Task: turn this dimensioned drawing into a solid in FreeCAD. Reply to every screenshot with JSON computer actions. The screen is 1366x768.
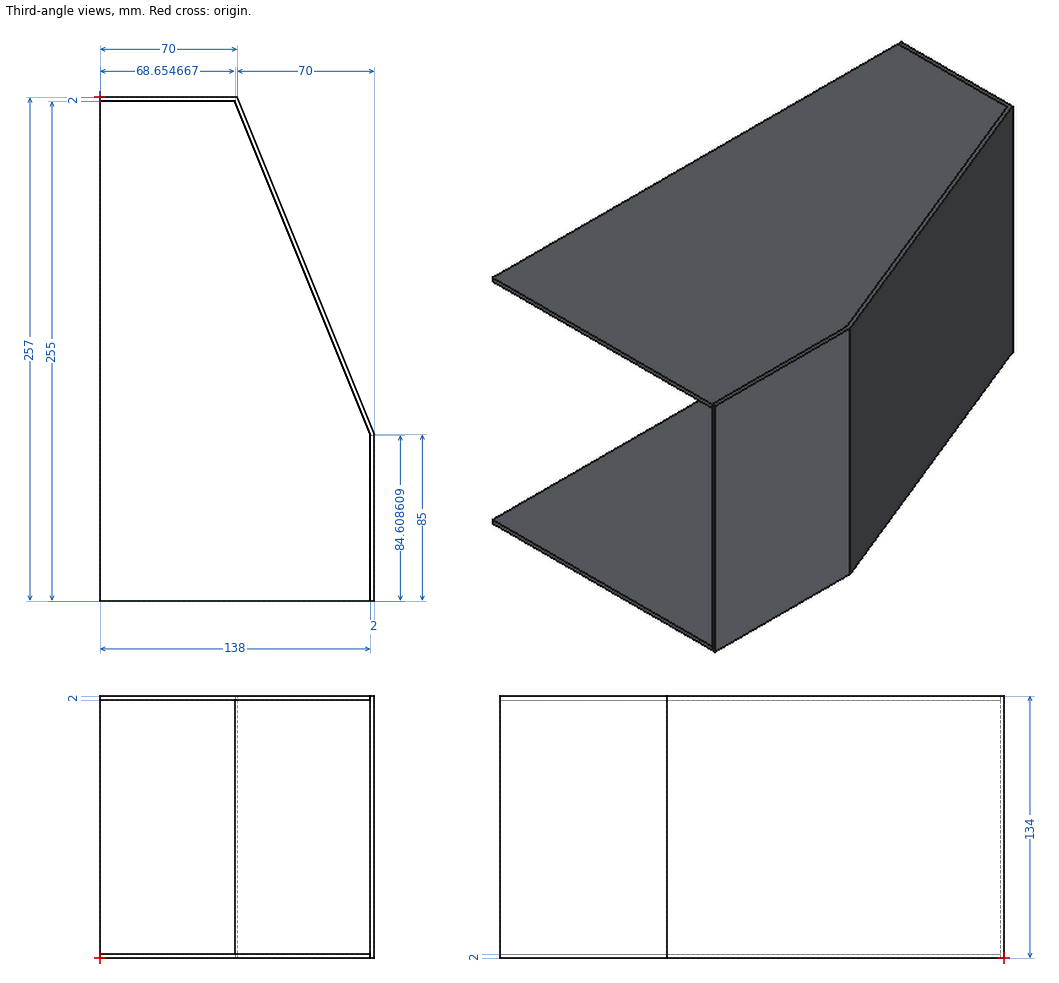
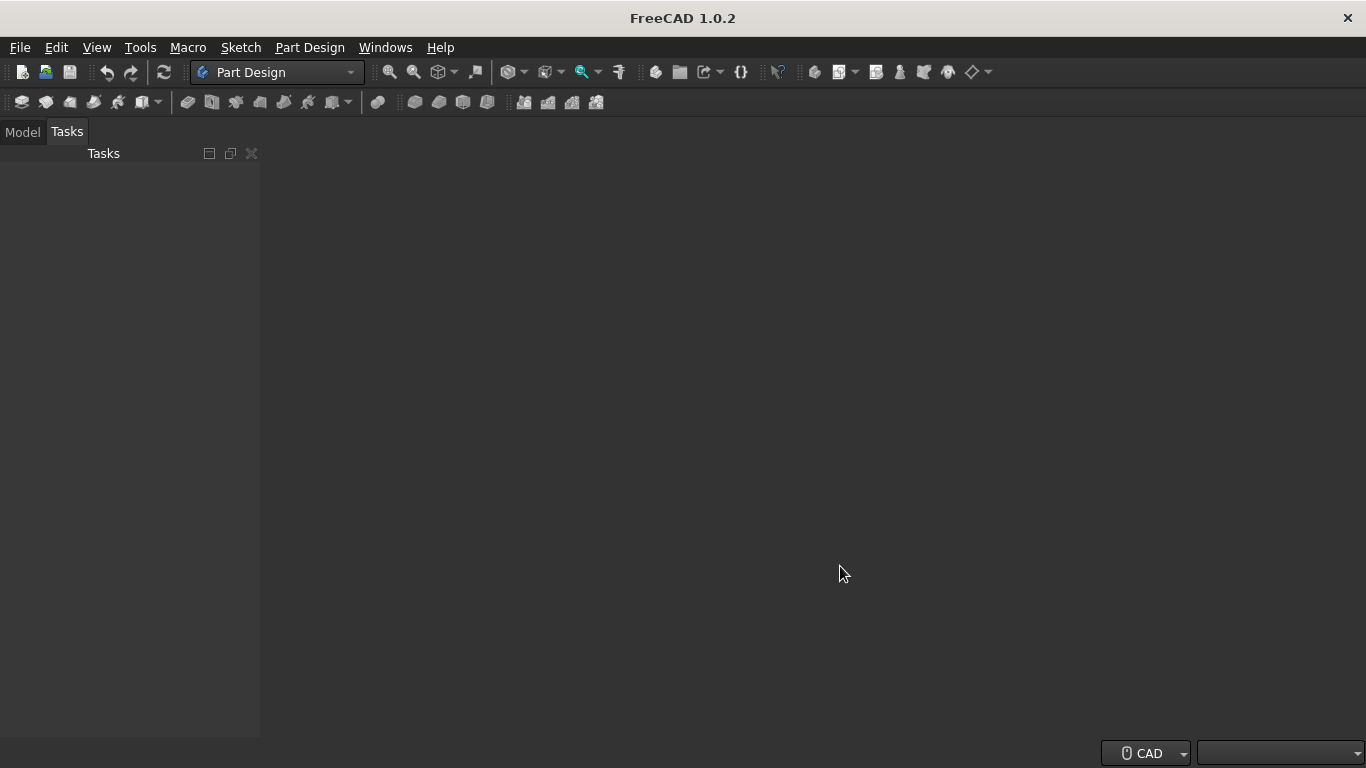
{"action": "left_click", "coordinate": [22, 72]}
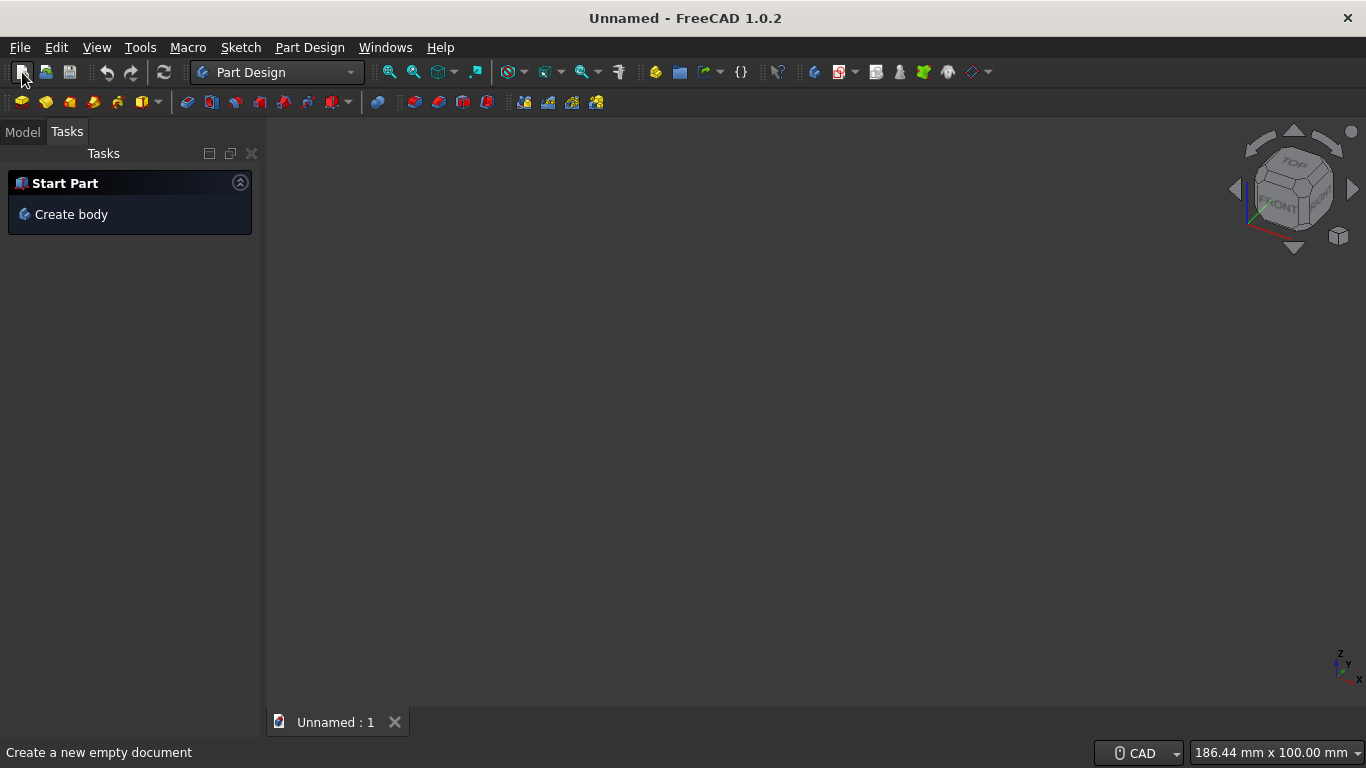
{"action": "left_click", "coordinate": [840, 72]}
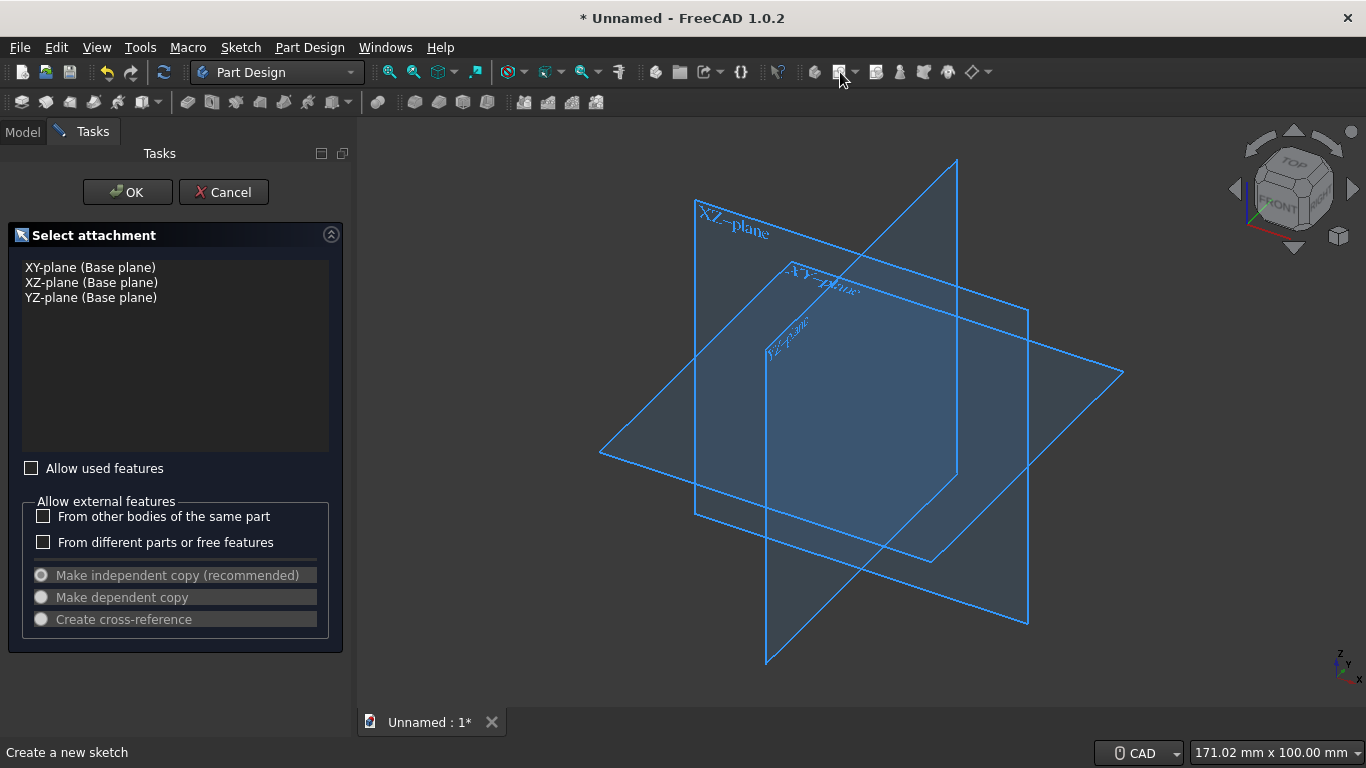
{"action": "left_click", "coordinate": [82, 268]}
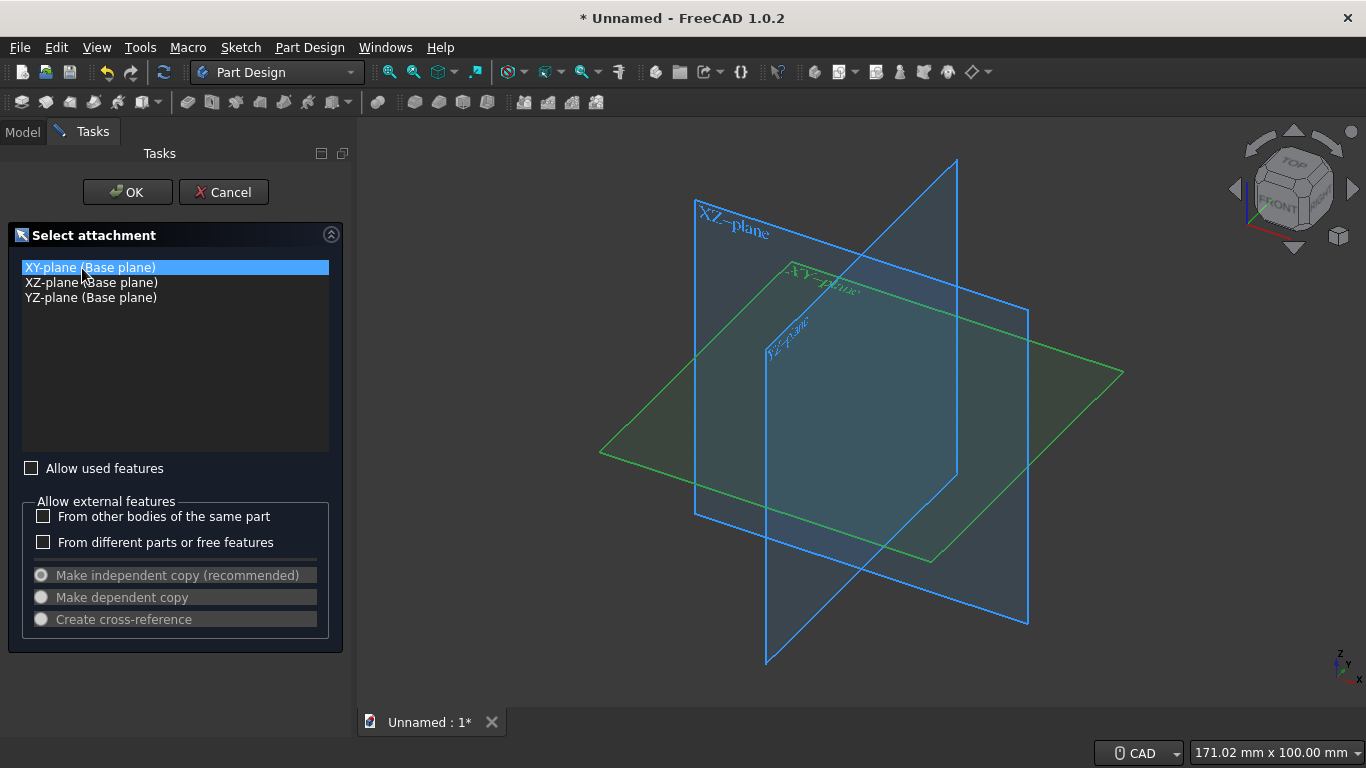
{"action": "left_click", "coordinate": [128, 192]}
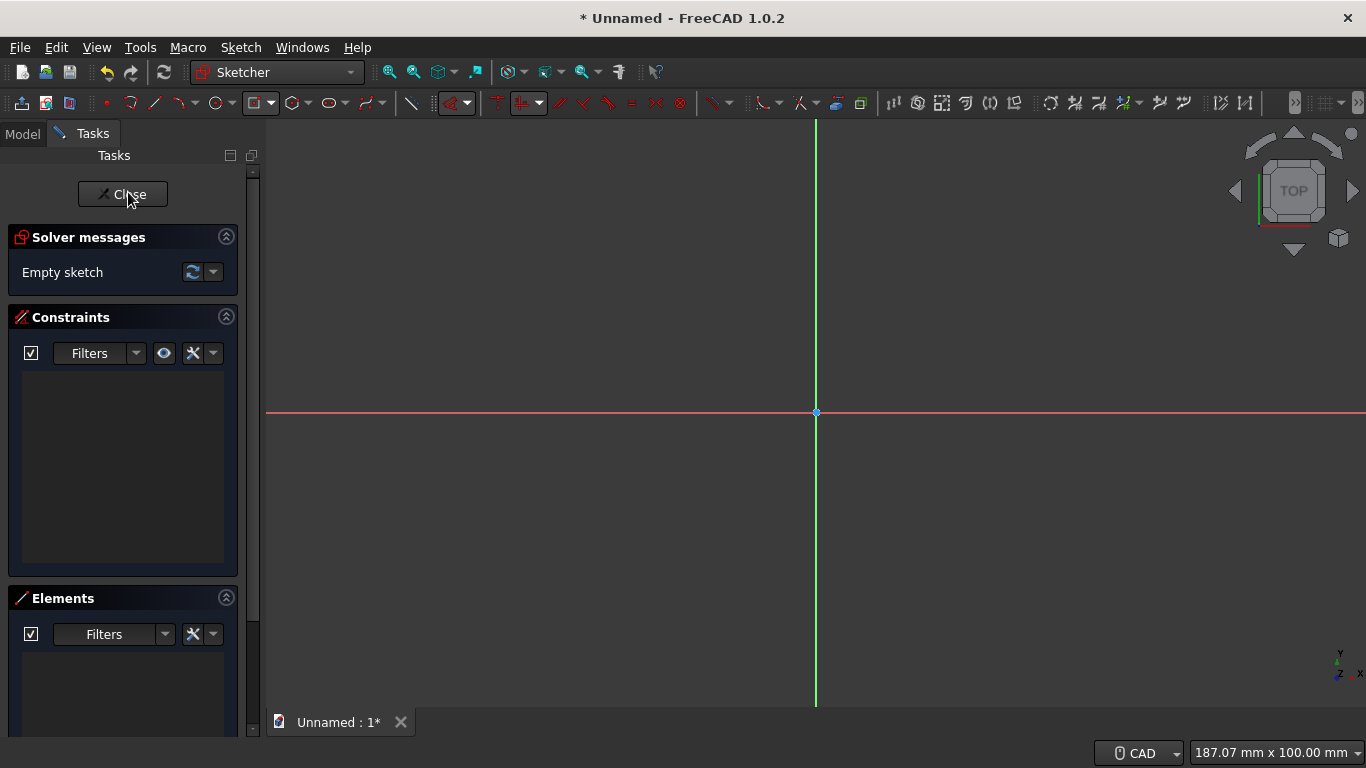
{"action": "scroll", "coordinate": [590, 166], "scroll_direction": "down", "scroll_amount": 7}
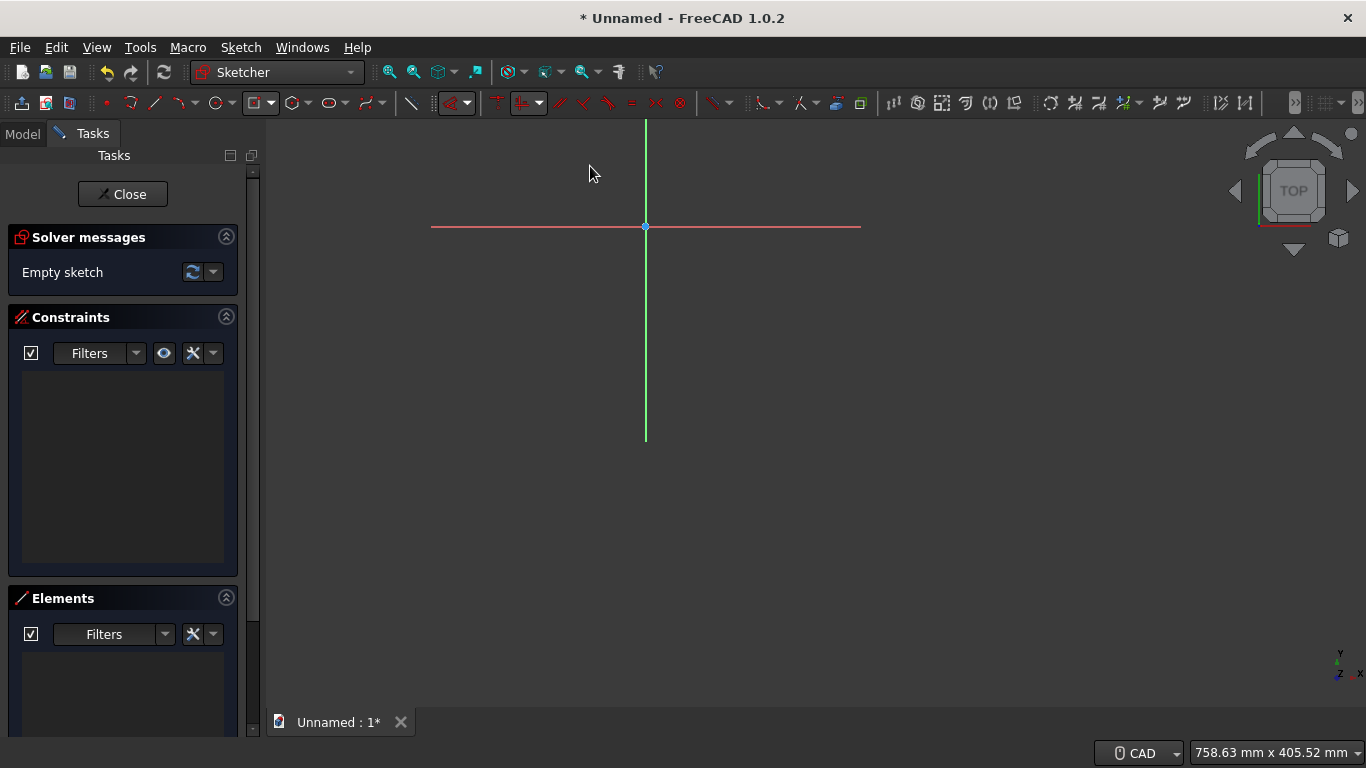
{"action": "key", "text": "g m"}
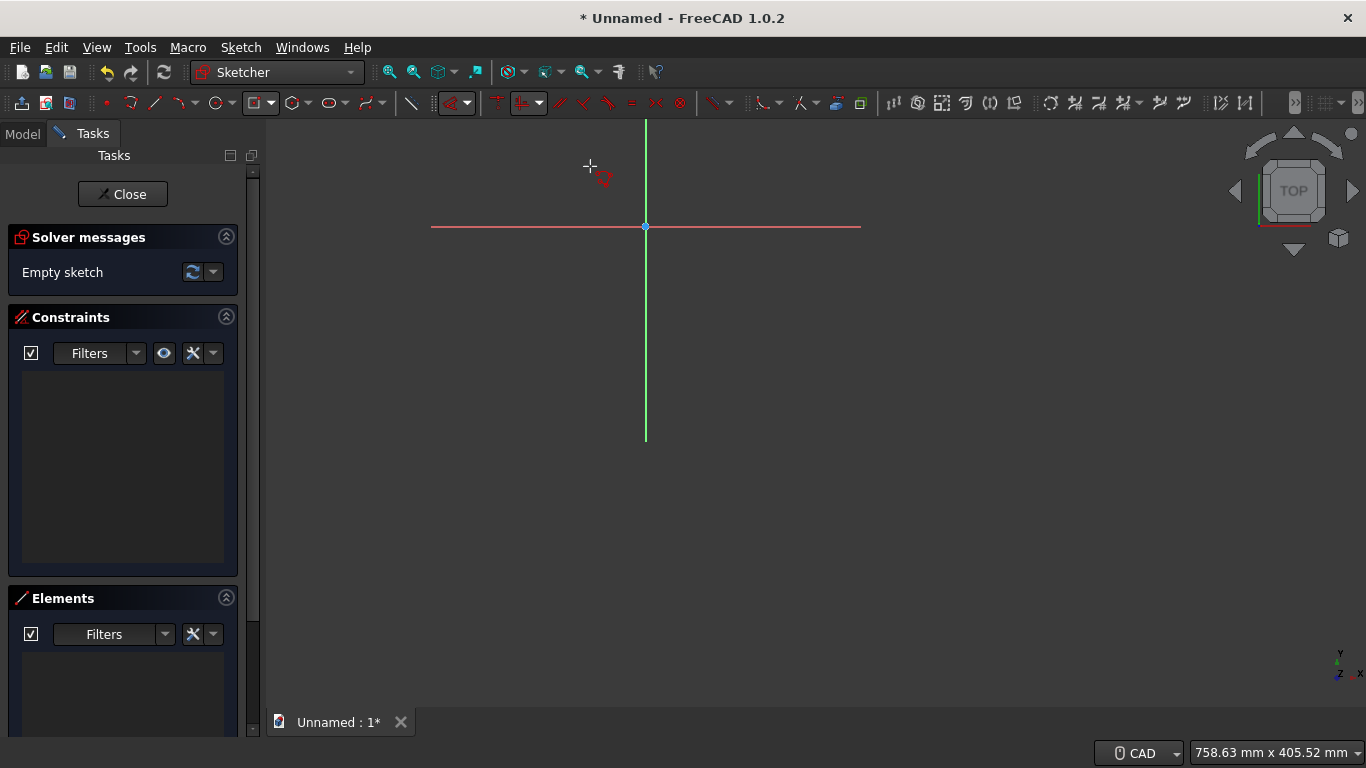
{"action": "left_click", "coordinate": [646, 227]}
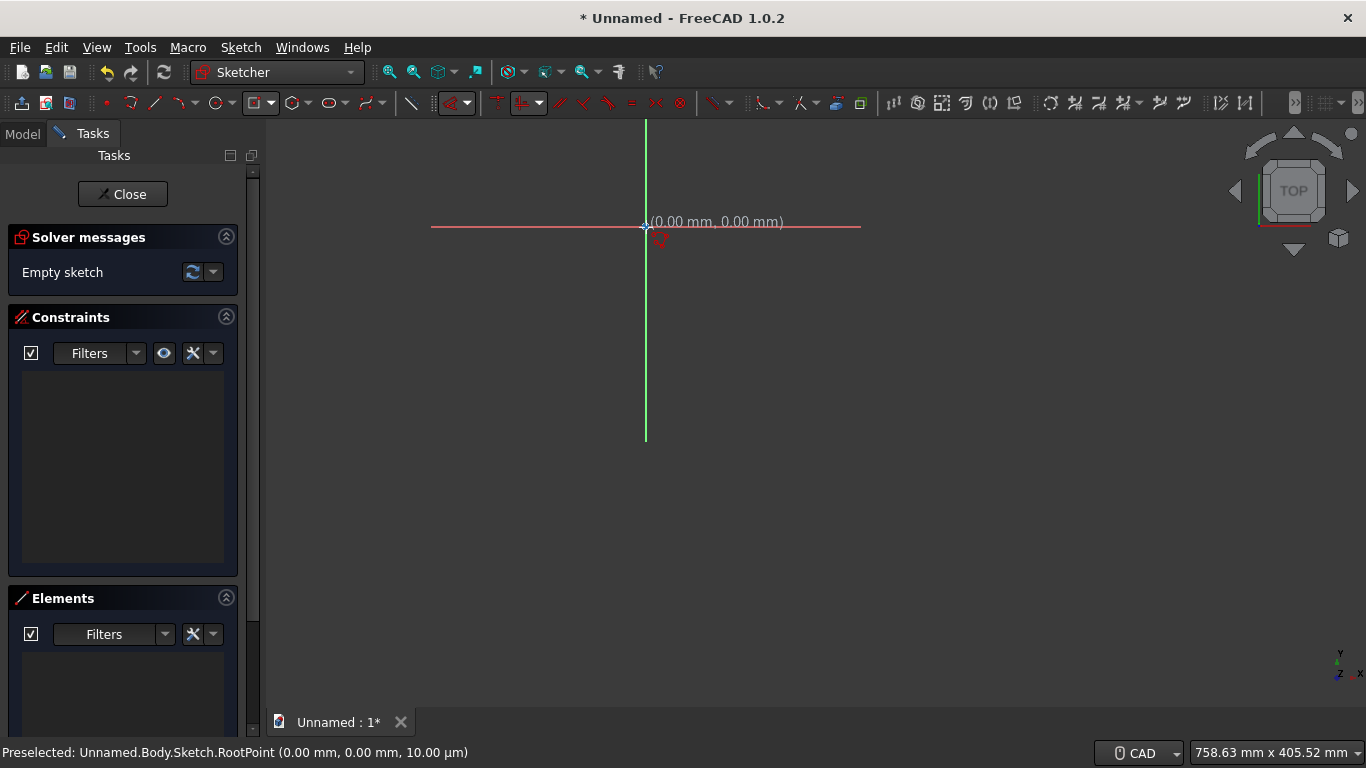
{"action": "scroll", "coordinate": [646, 230], "scroll_direction": "up", "scroll_amount": 9}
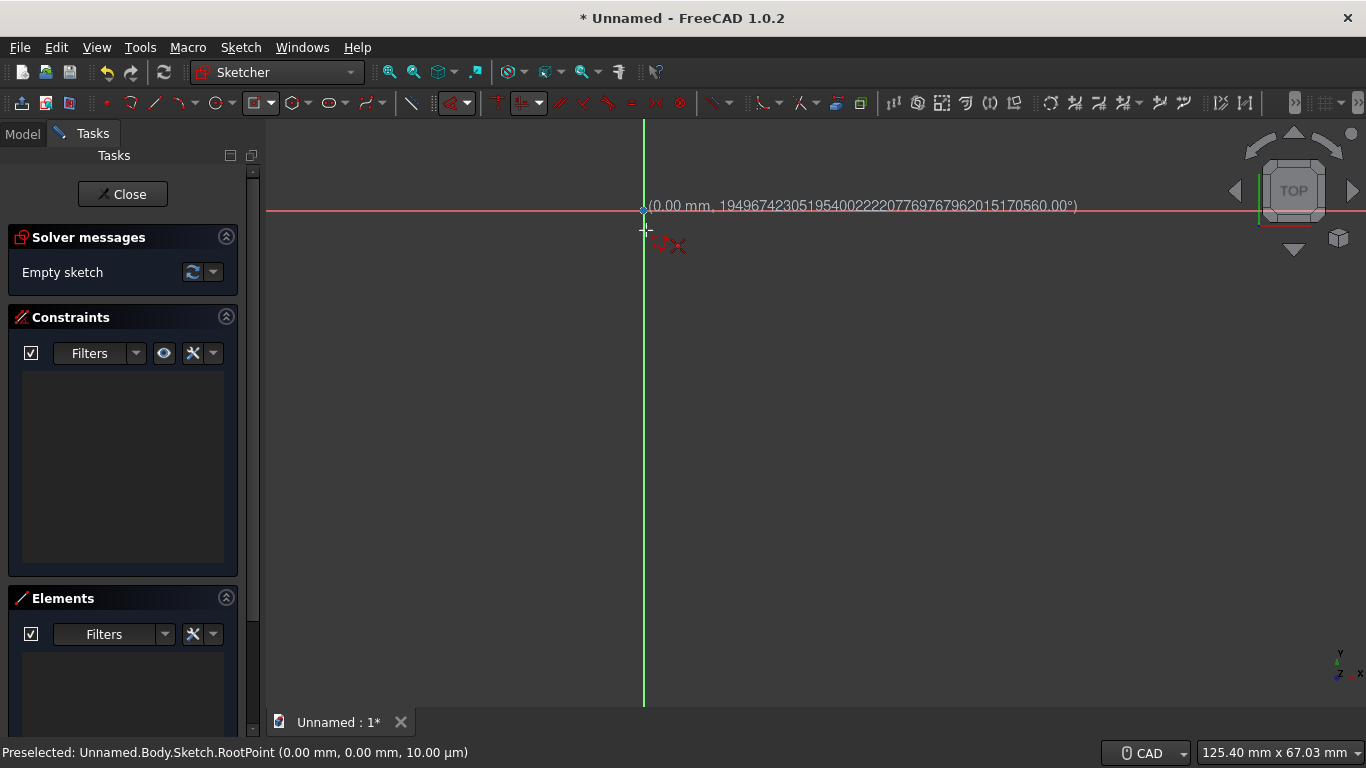
{"action": "left_click", "coordinate": [653, 228]}